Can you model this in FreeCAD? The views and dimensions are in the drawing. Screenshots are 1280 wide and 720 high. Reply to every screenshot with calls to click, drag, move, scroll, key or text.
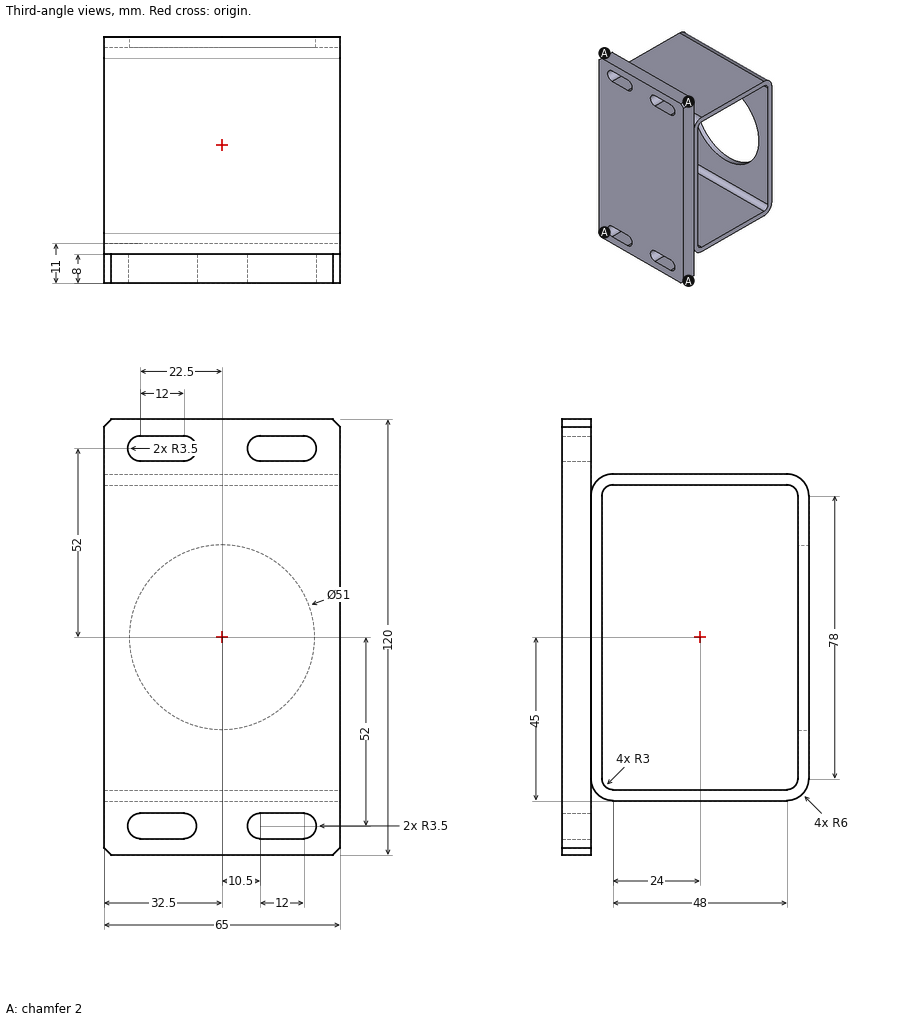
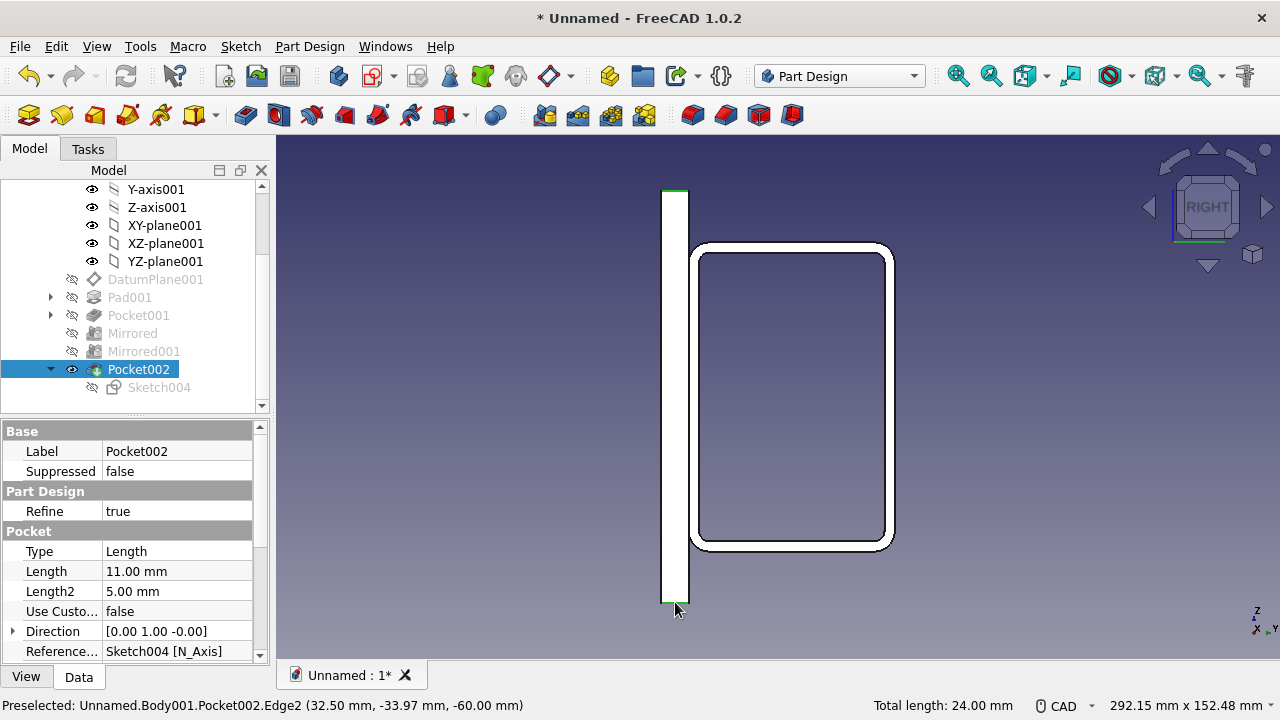
key(5)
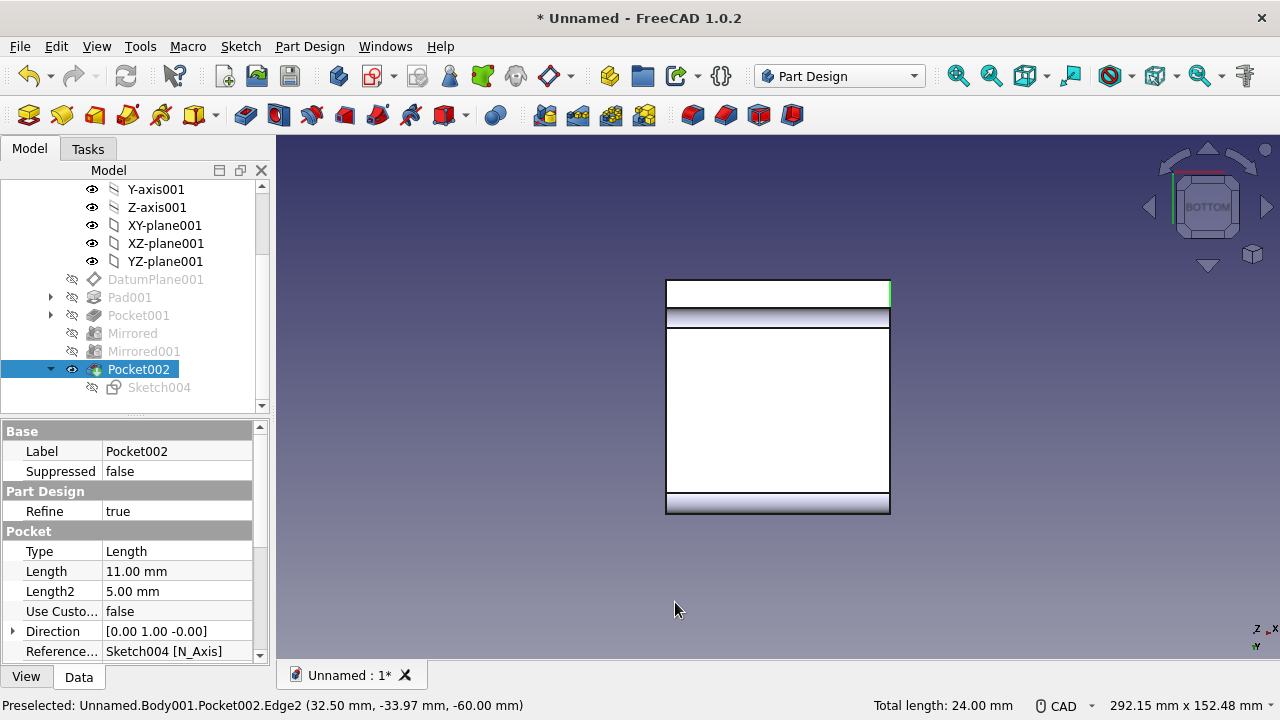
click(959, 76)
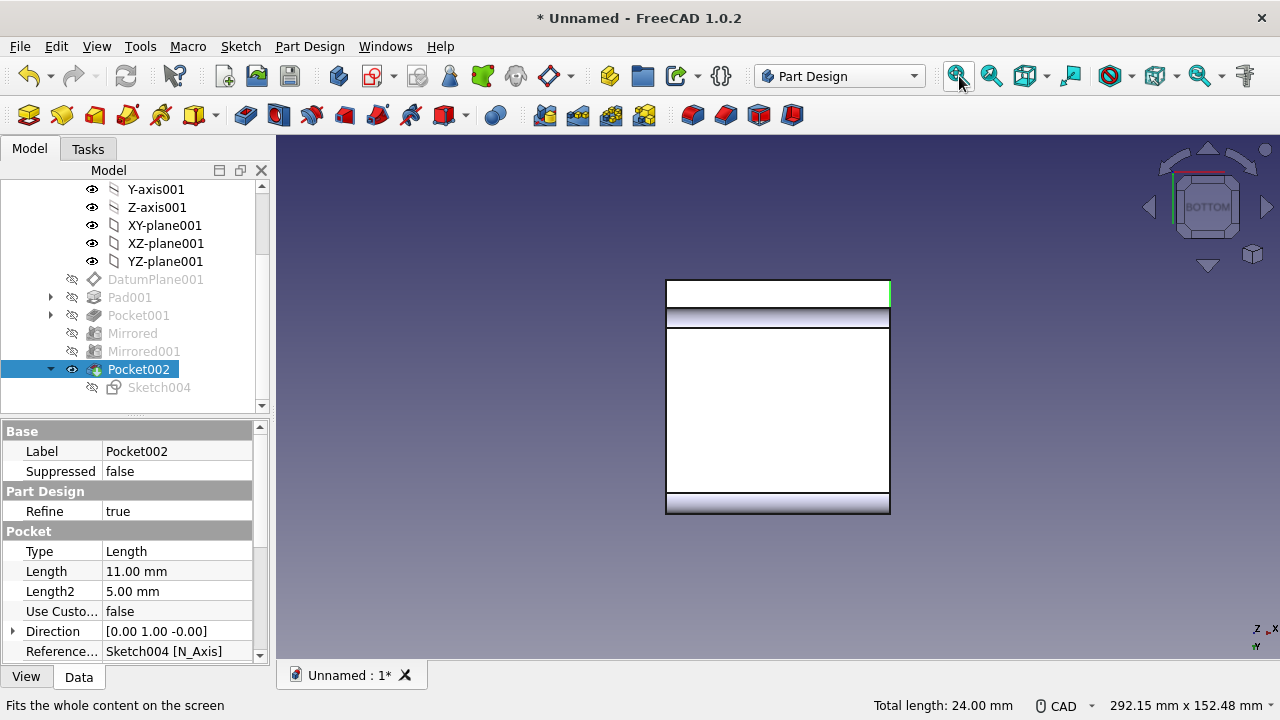
click(666, 293, ctrl)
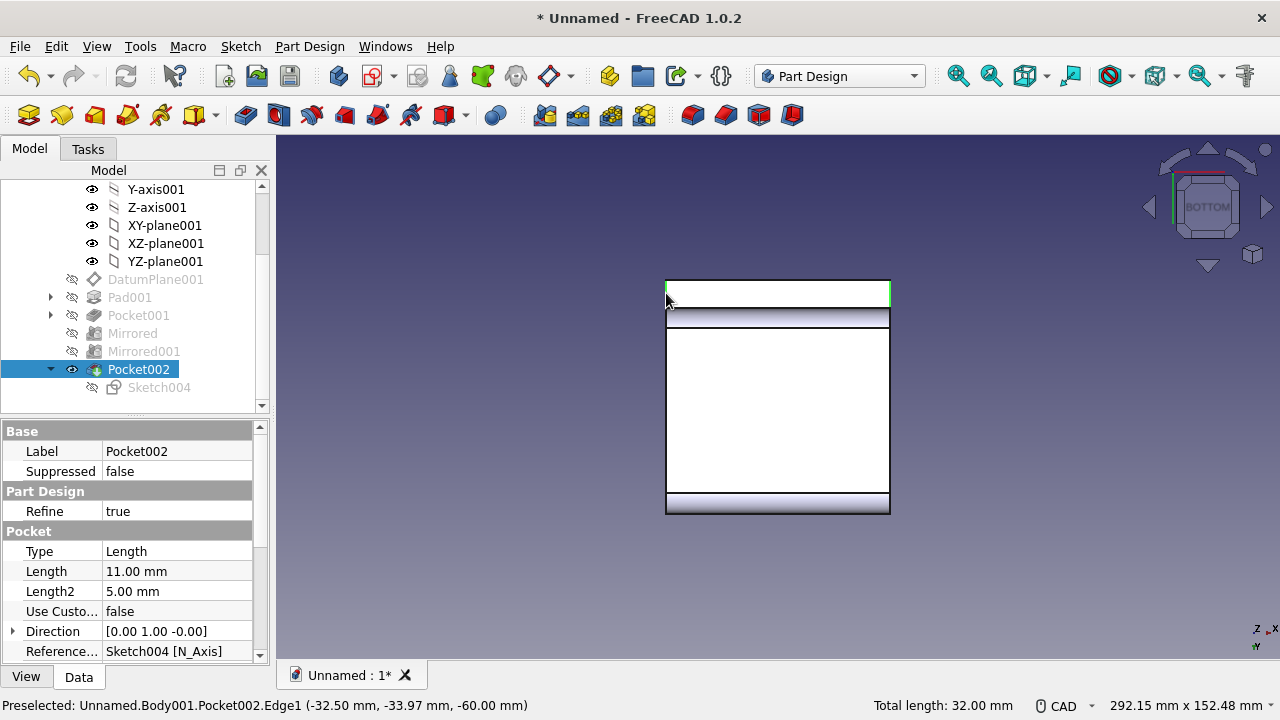
click(726, 116)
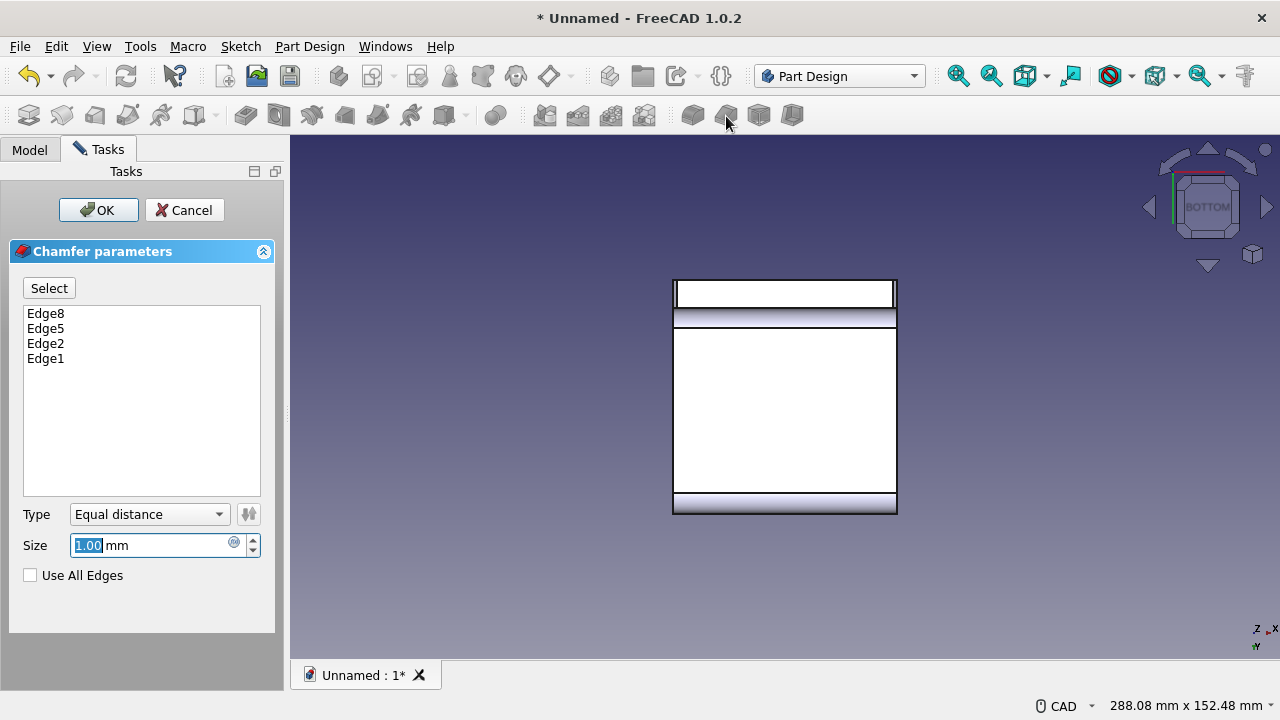
text(2)
key(Tab)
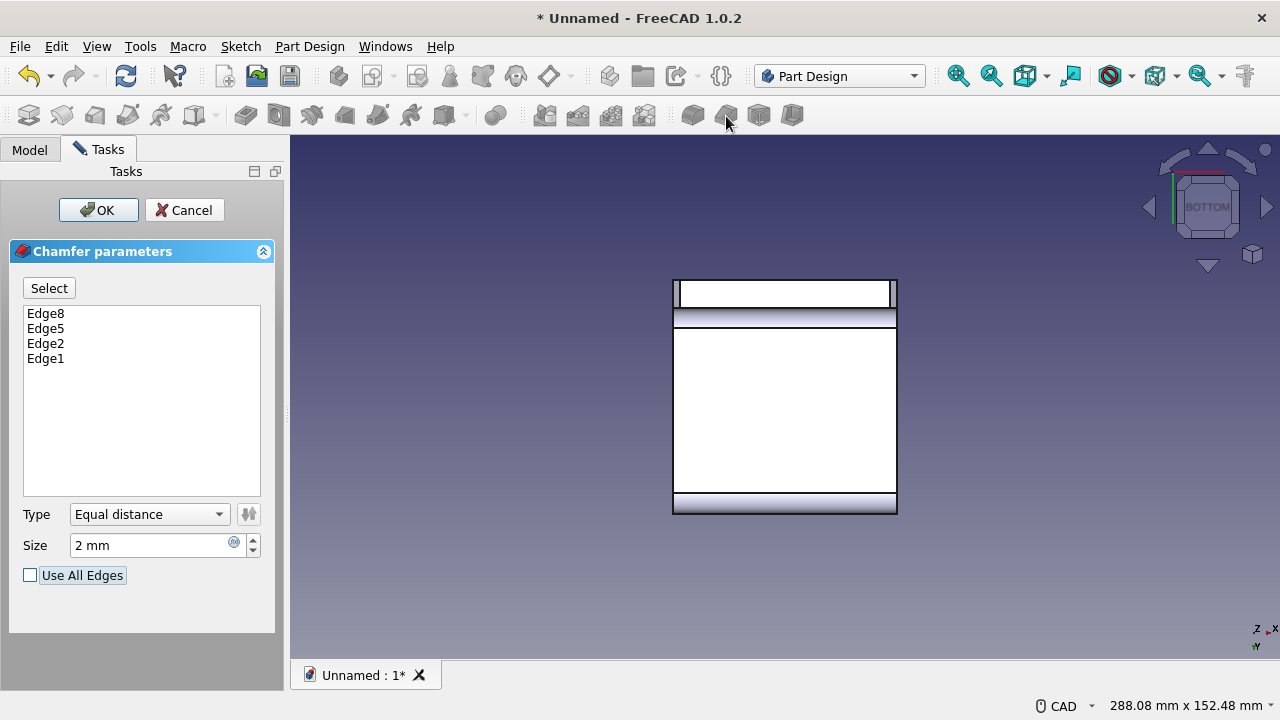
click(99, 210)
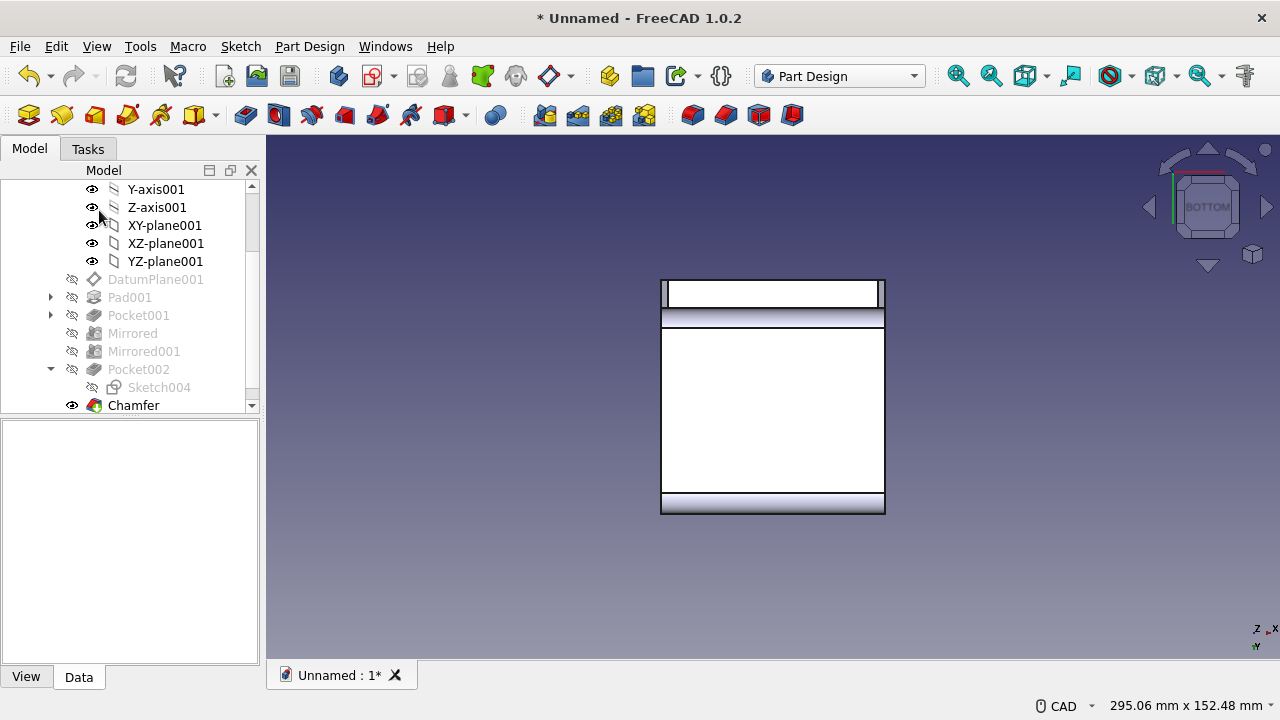
key(0)